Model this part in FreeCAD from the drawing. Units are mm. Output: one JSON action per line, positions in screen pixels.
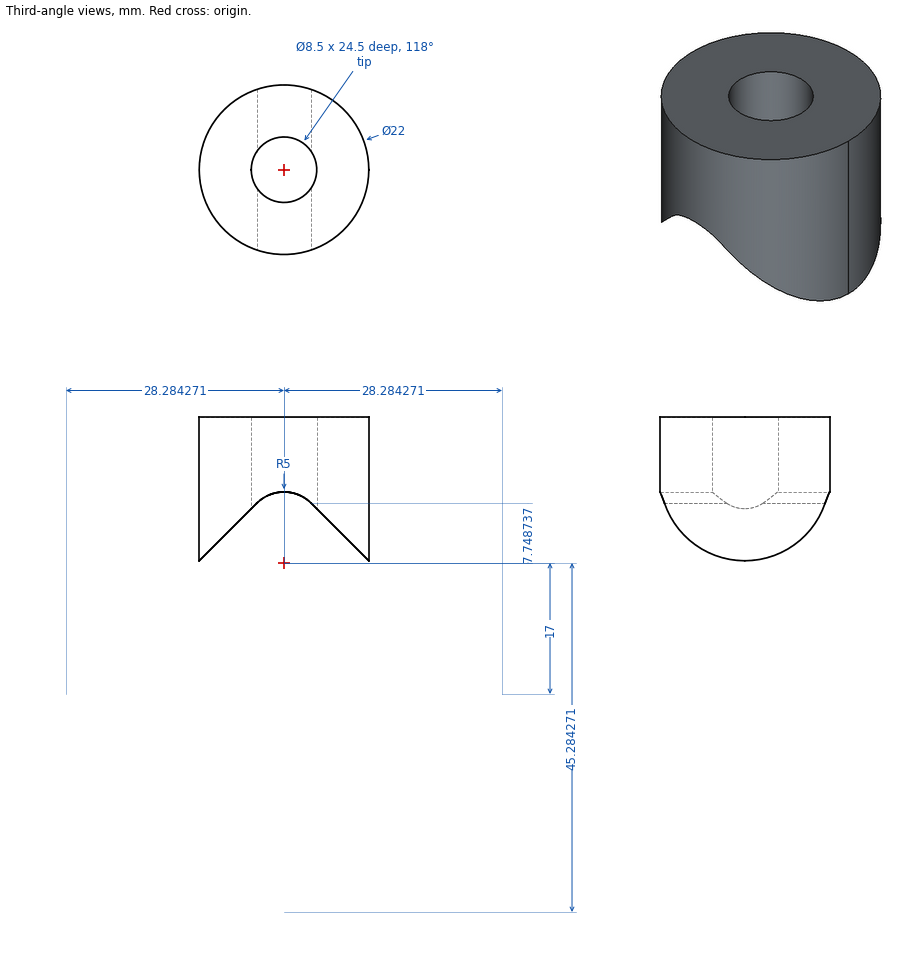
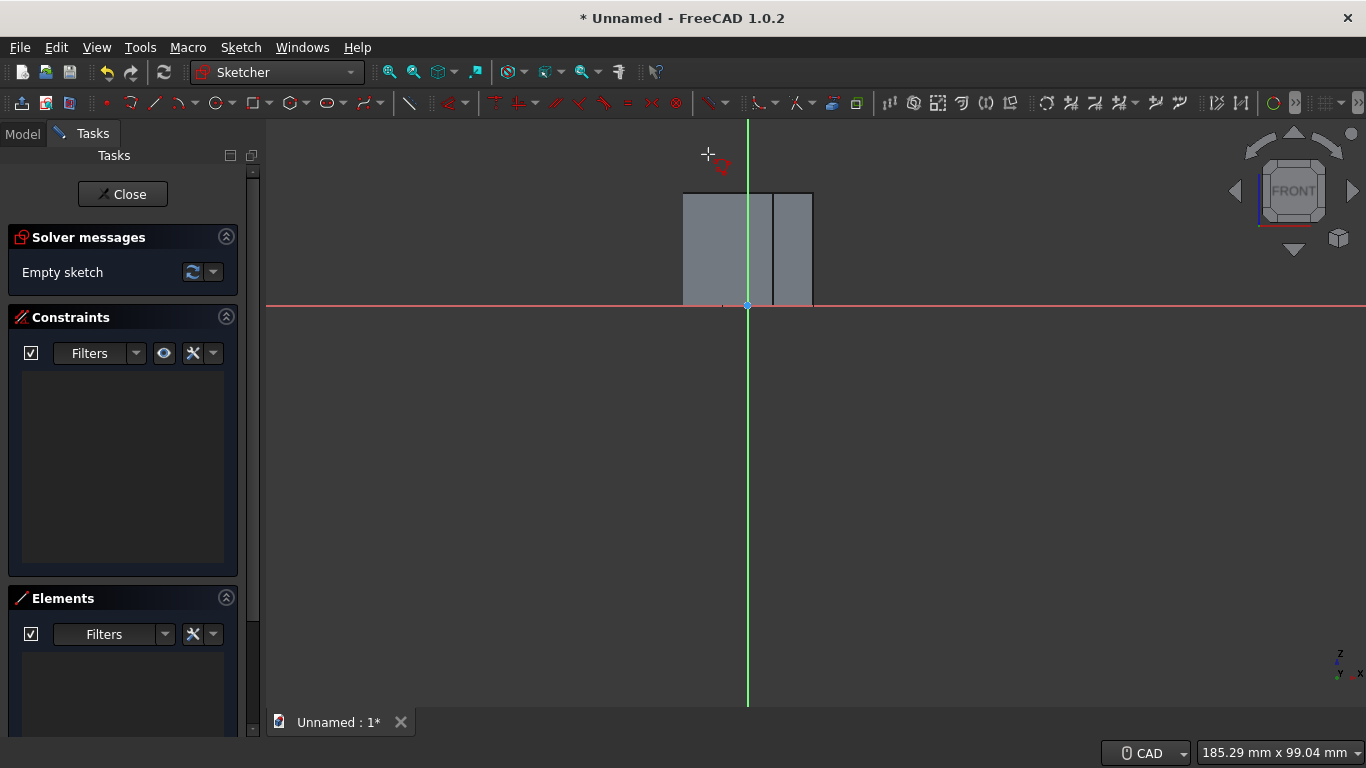
{"action": "left_click", "coordinate": [769, 260]}
{"action": "left_click", "coordinate": [916, 407]}
{"action": "left_click", "coordinate": [748, 575]}
{"action": "left_click", "coordinate": [580, 407]}
{"action": "left_click", "coordinate": [727, 260]}
{"action": "right_click", "coordinate": [727, 260]}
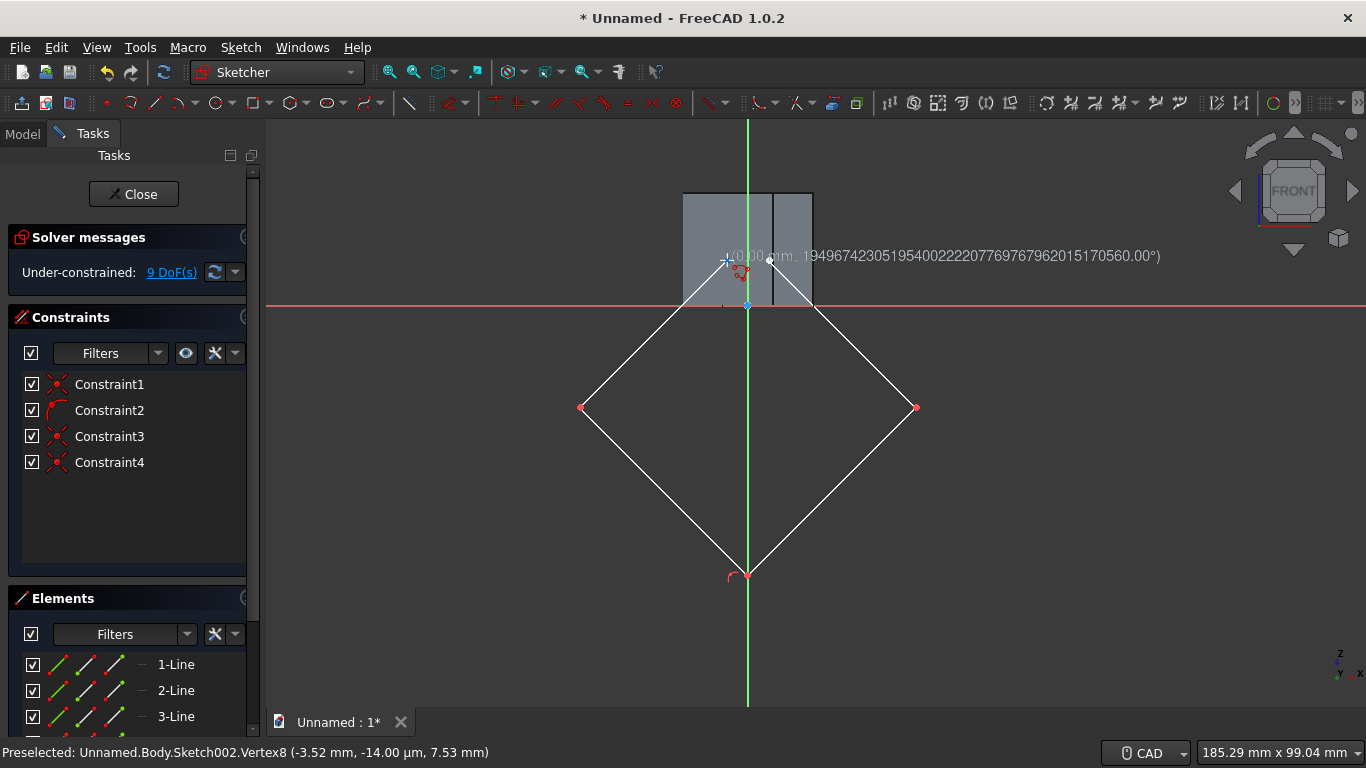
{"action": "key", "text": "g 3 a"}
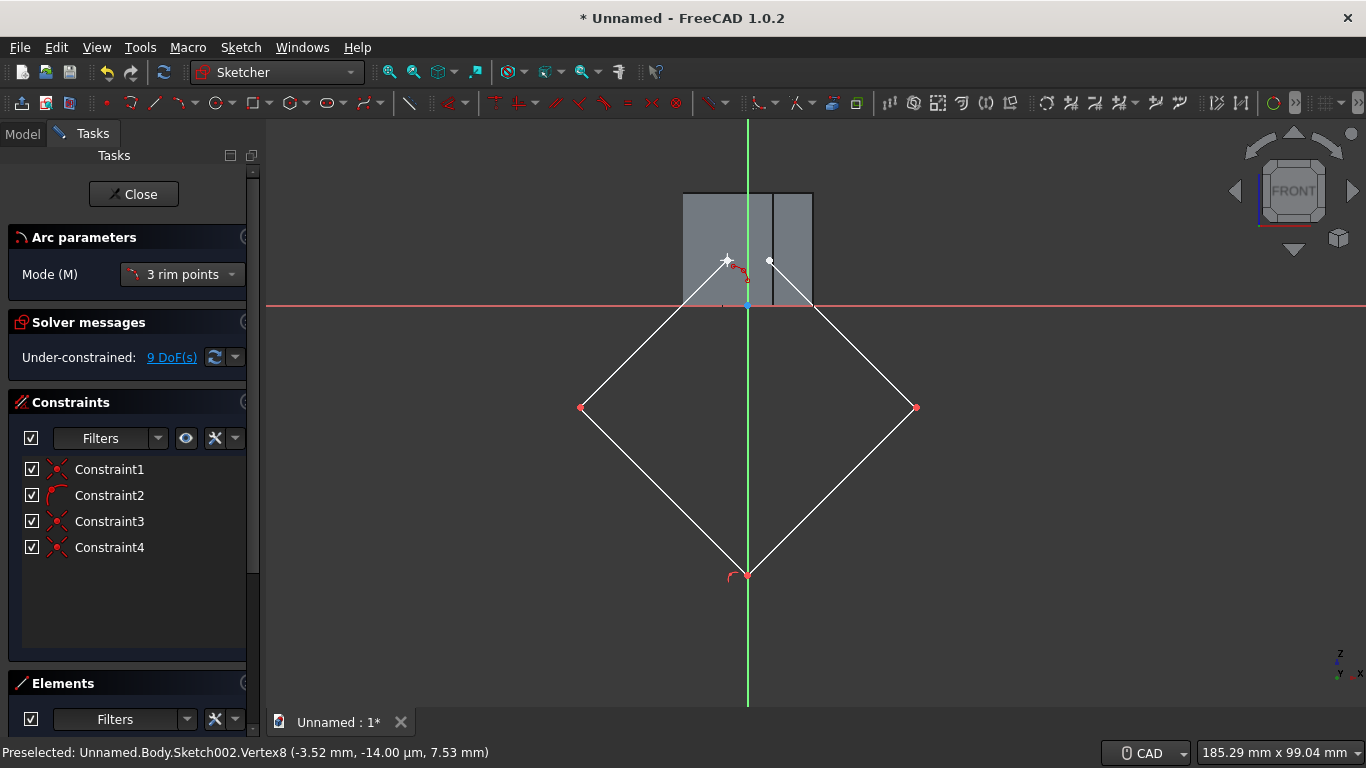
{"action": "left_click", "coordinate": [727, 261]}
{"action": "left_click", "coordinate": [769, 261]}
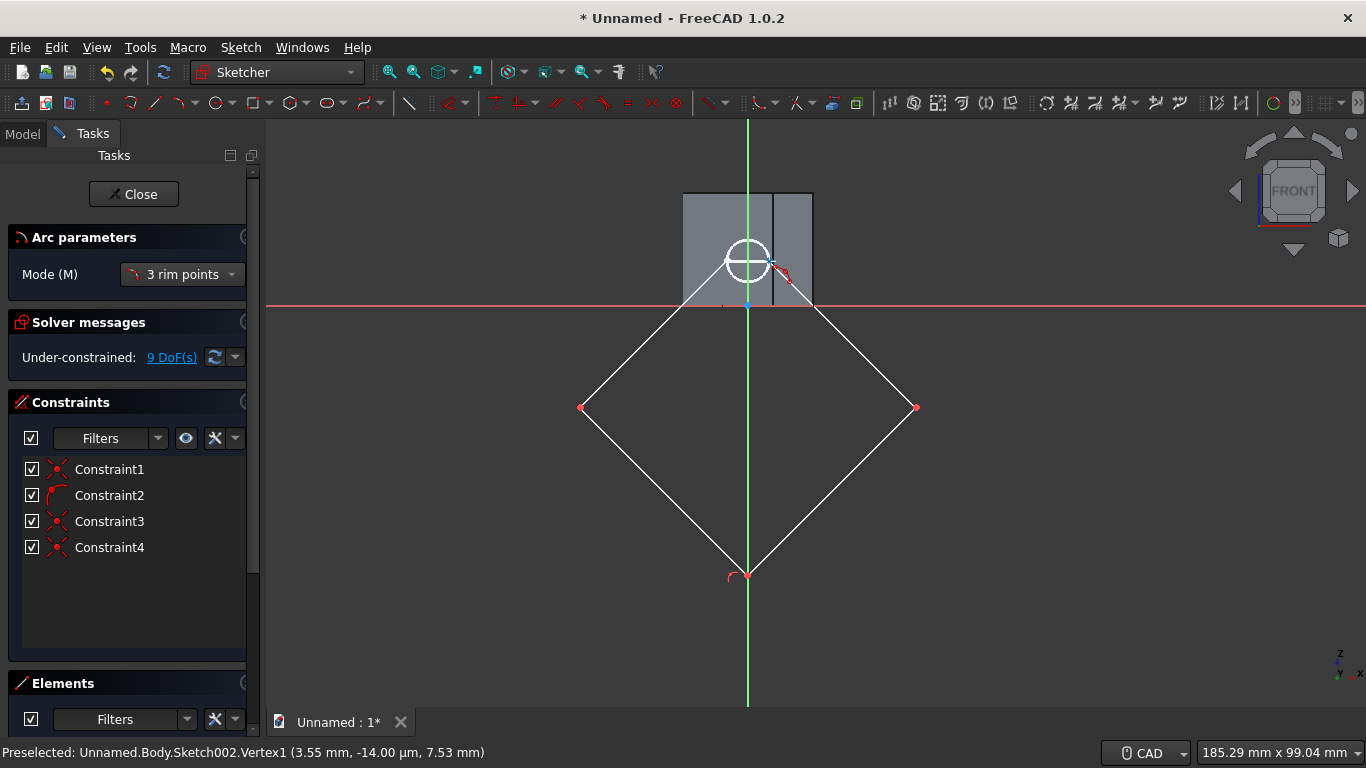
{"action": "scroll", "coordinate": [739, 252], "scroll_direction": "up", "scroll_amount": 4}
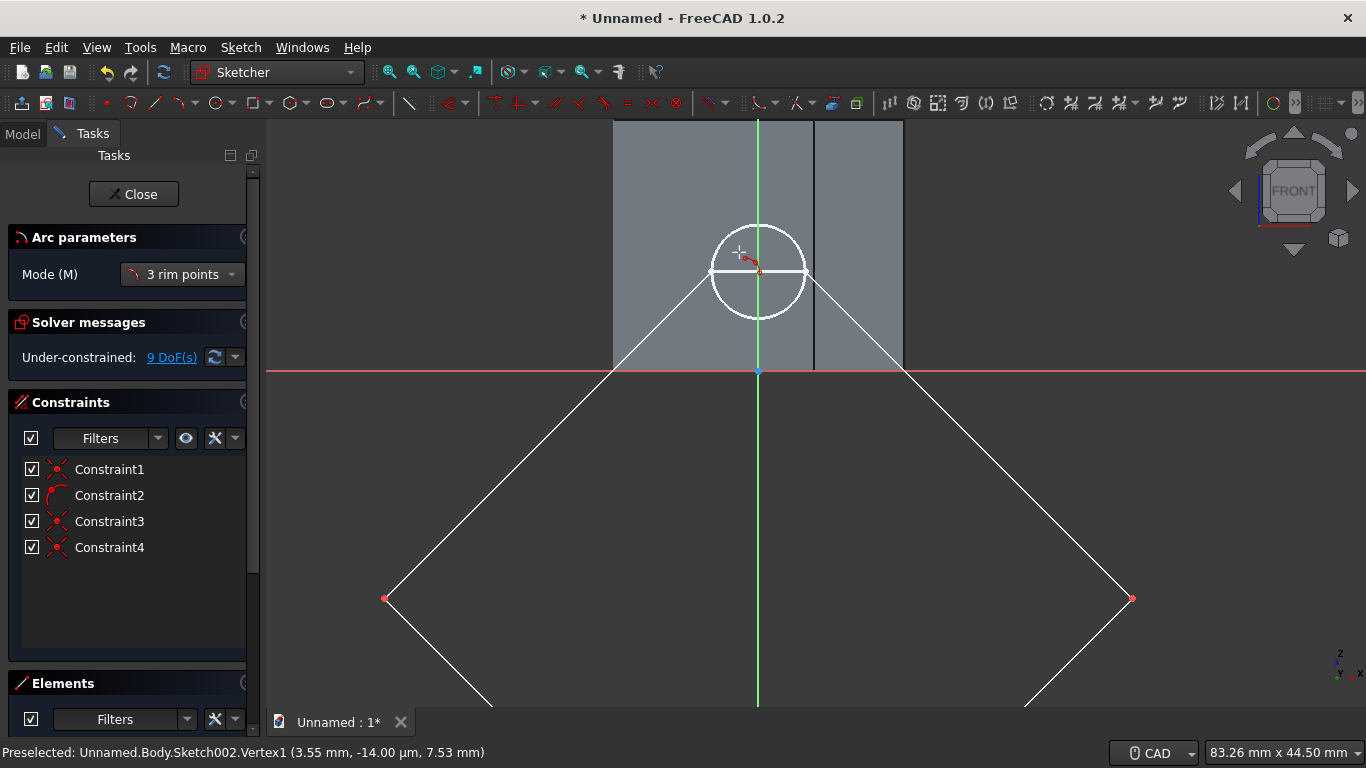
{"action": "left_click", "coordinate": [738, 253]}
{"action": "key", "text": "Escape"}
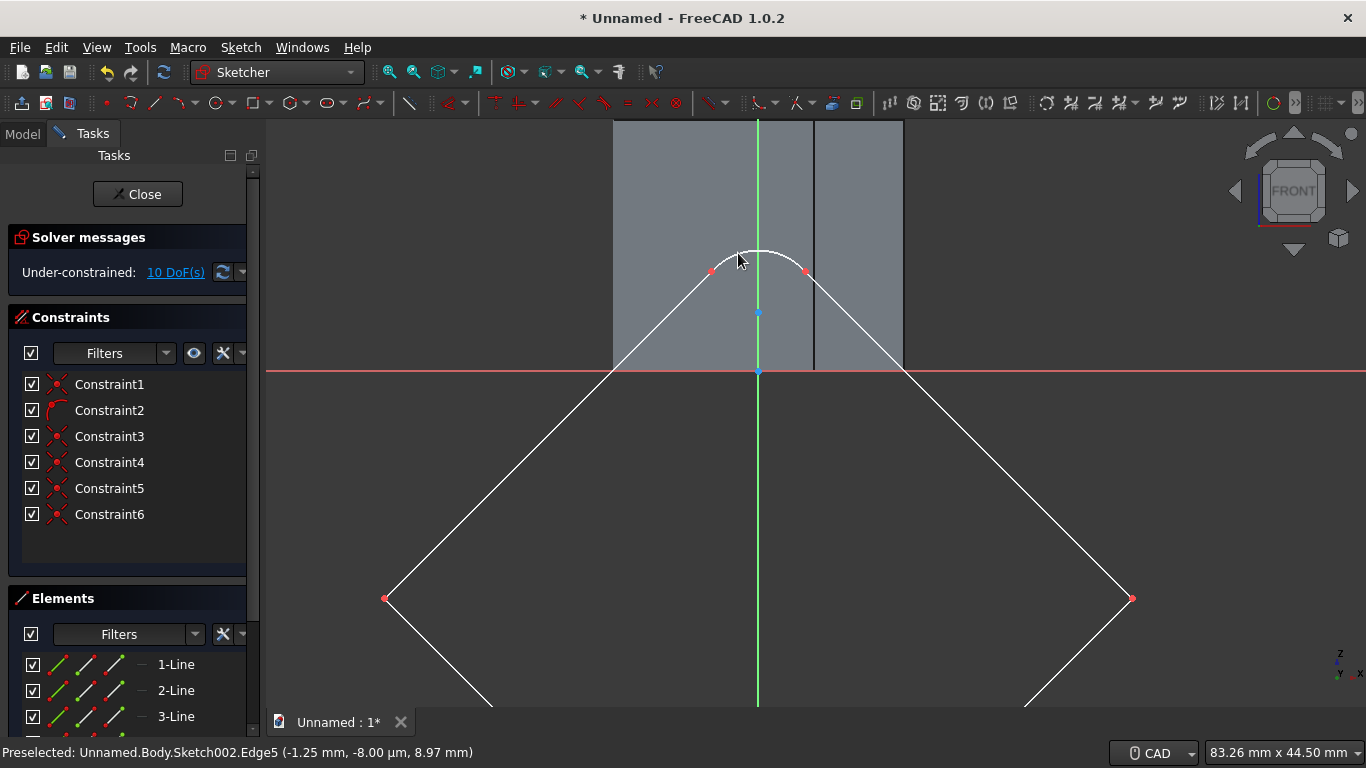
{"action": "left_click", "coordinate": [903, 370]}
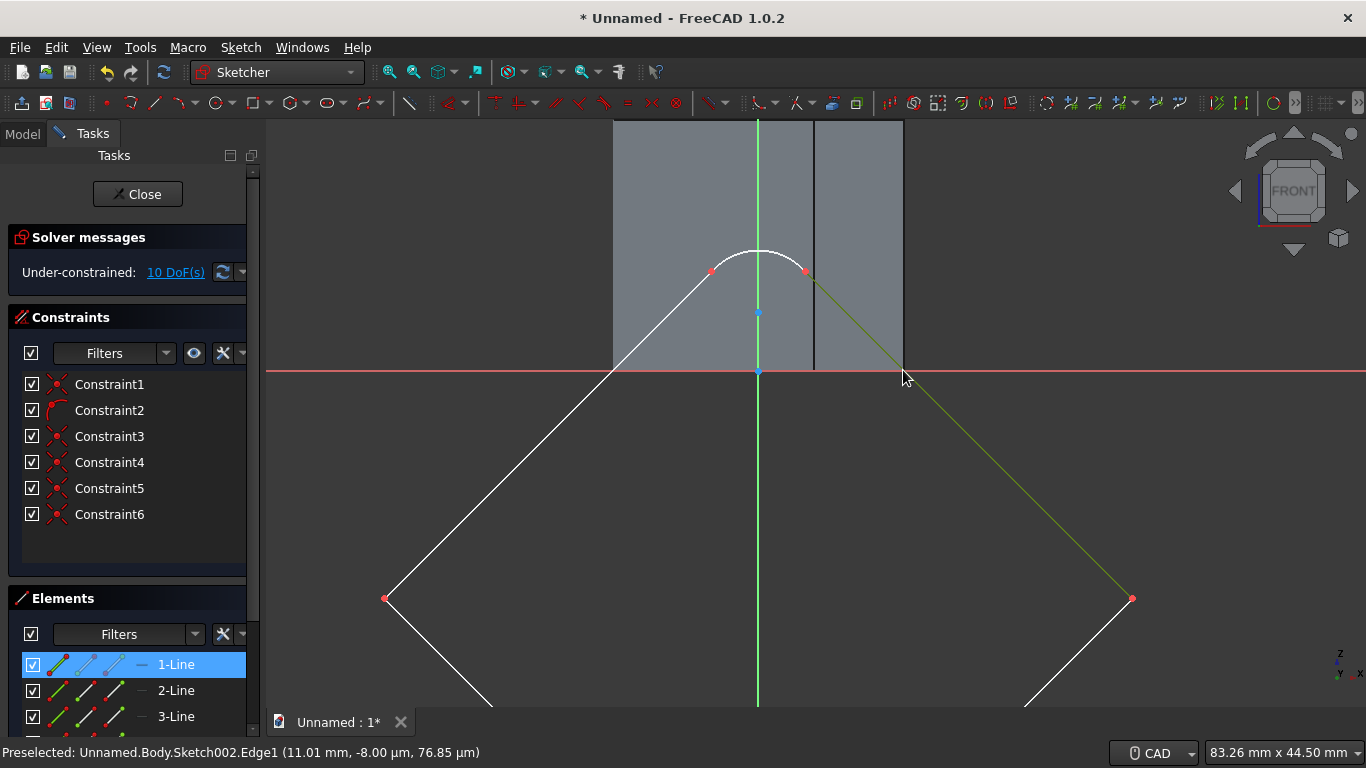
{"action": "left_click", "coordinate": [779, 254]}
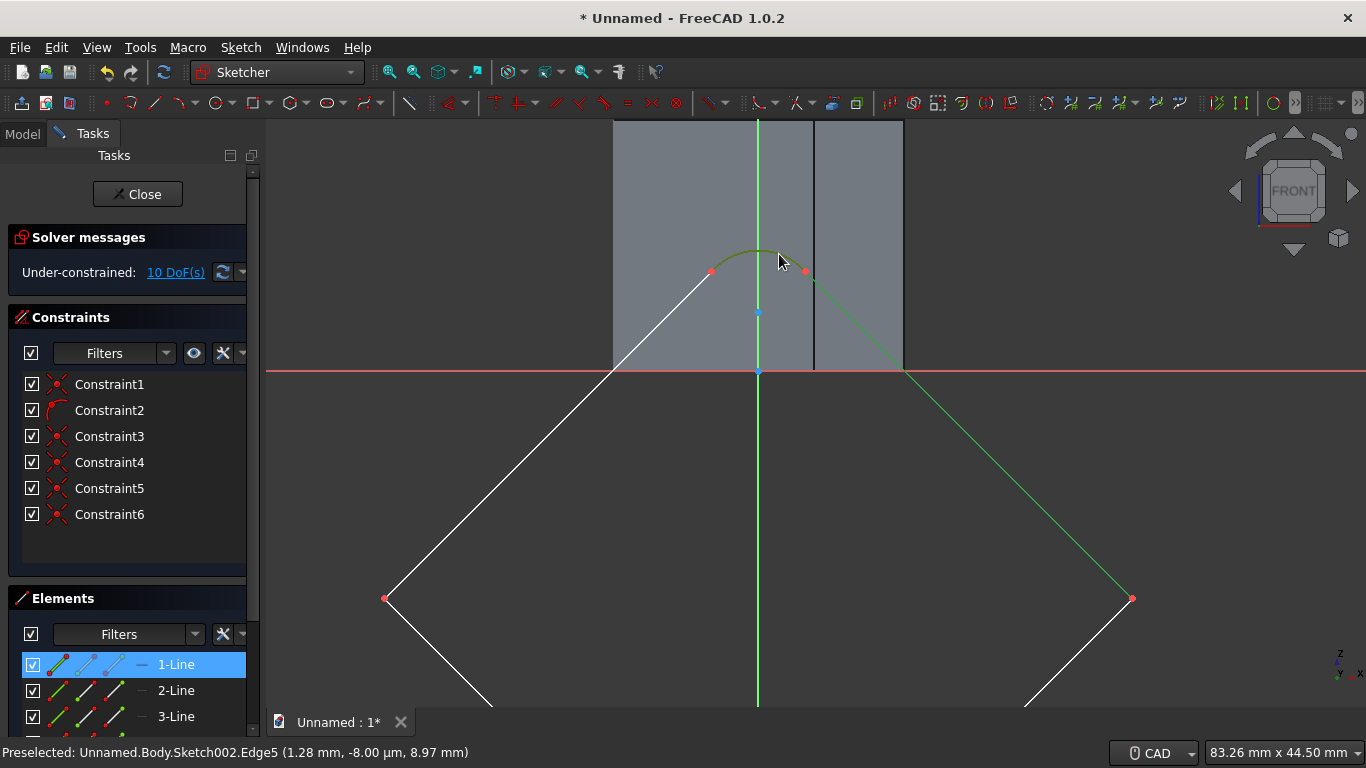
{"action": "key", "text": "t"}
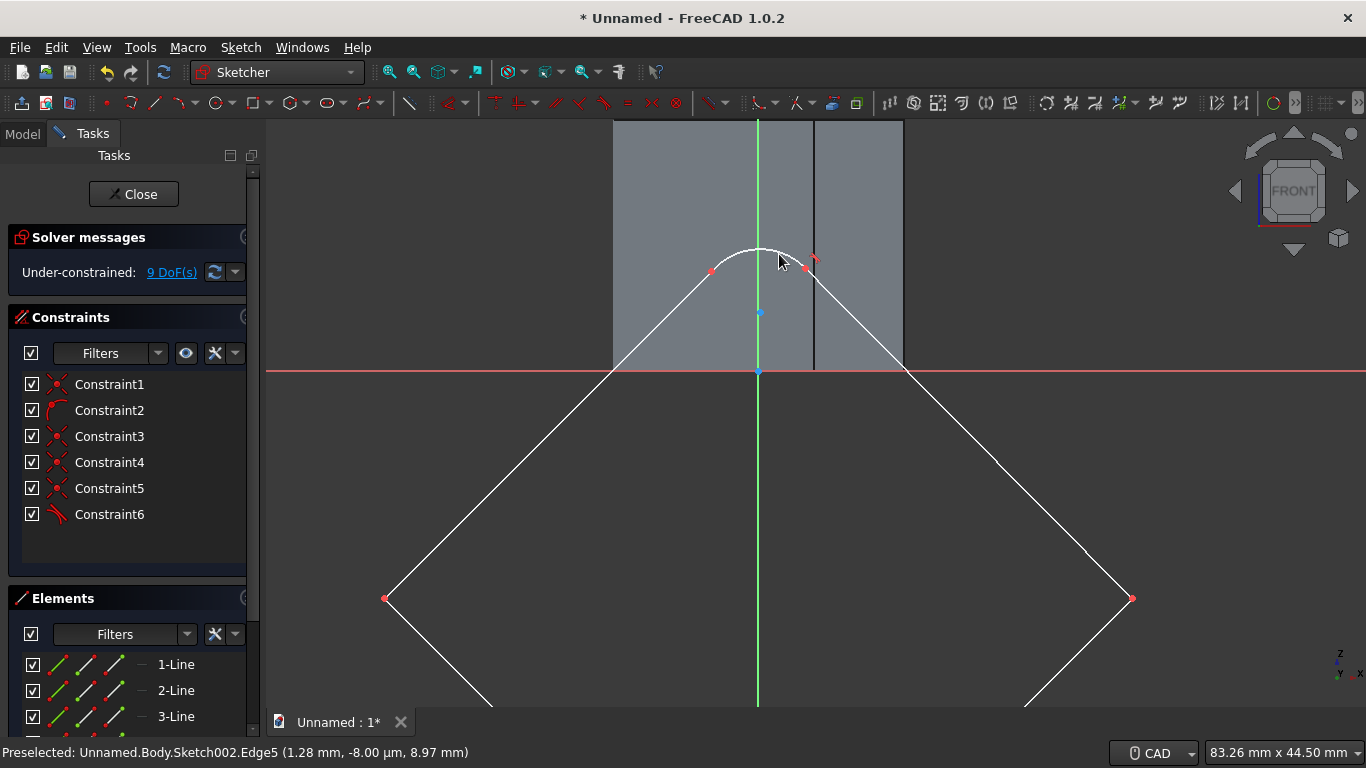
{"action": "left_click", "coordinate": [483, 501]}